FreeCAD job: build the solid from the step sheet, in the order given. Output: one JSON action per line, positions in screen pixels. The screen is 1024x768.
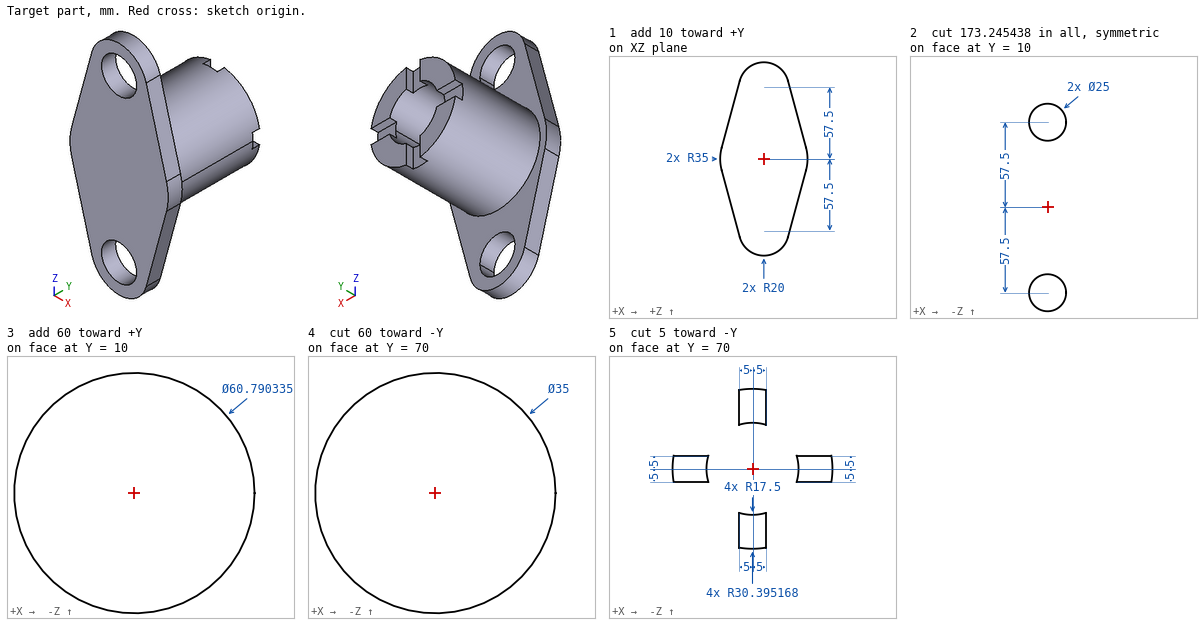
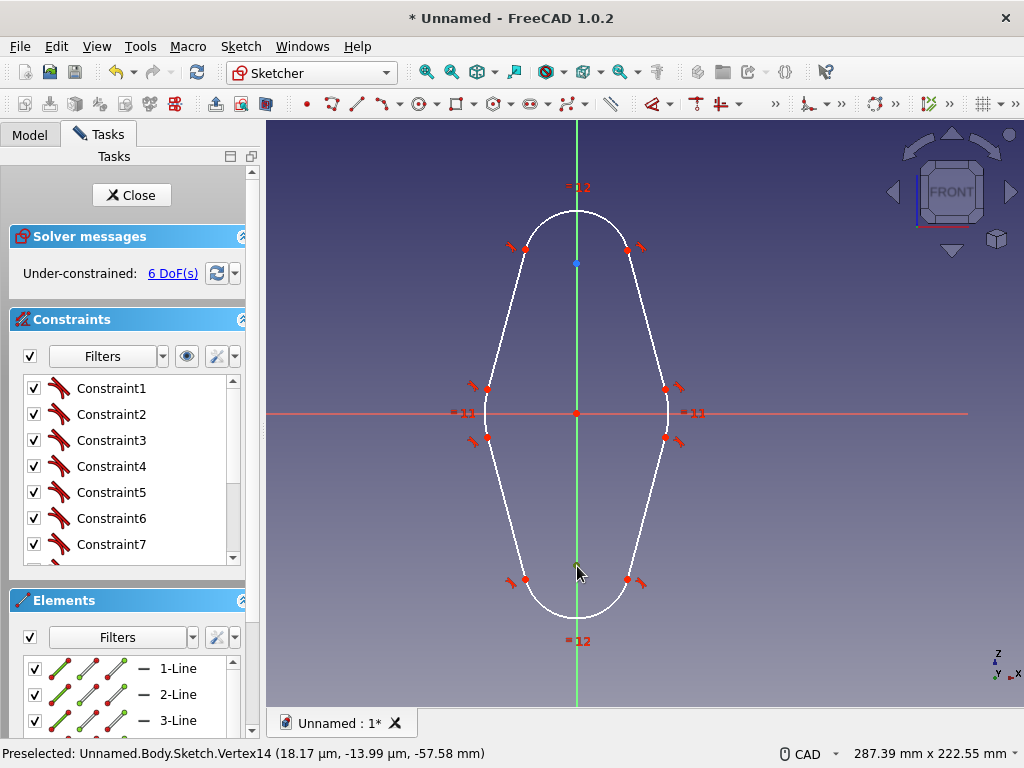
{"action": "left_click", "coordinate": [577, 527]}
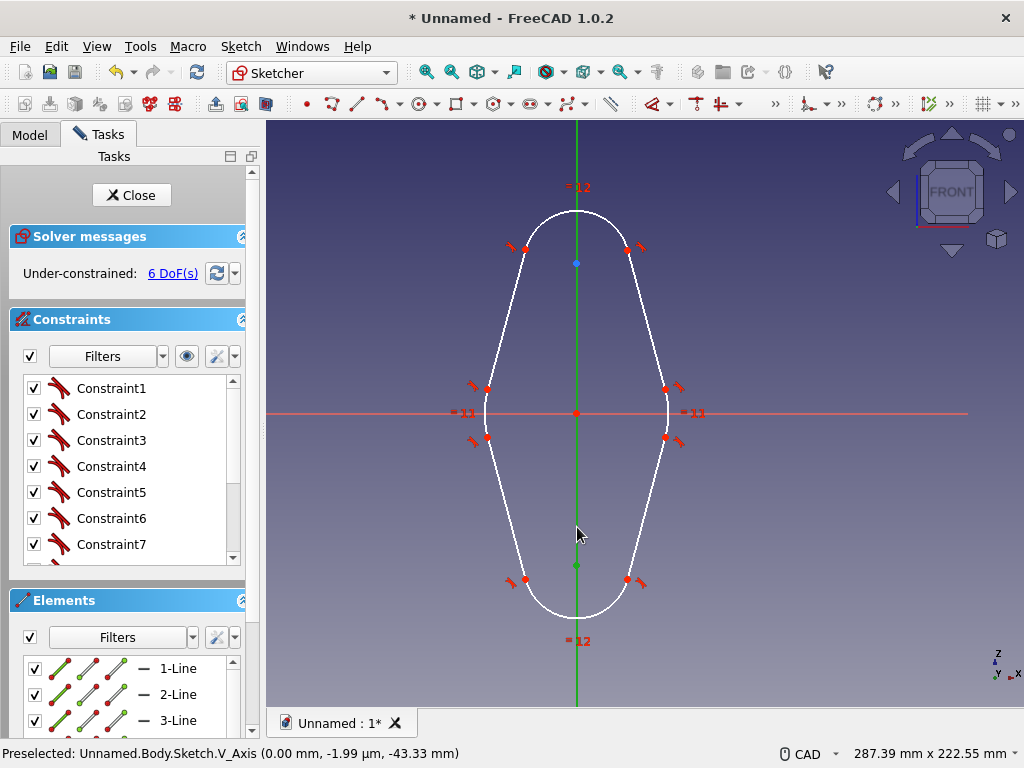
{"action": "key", "text": "c"}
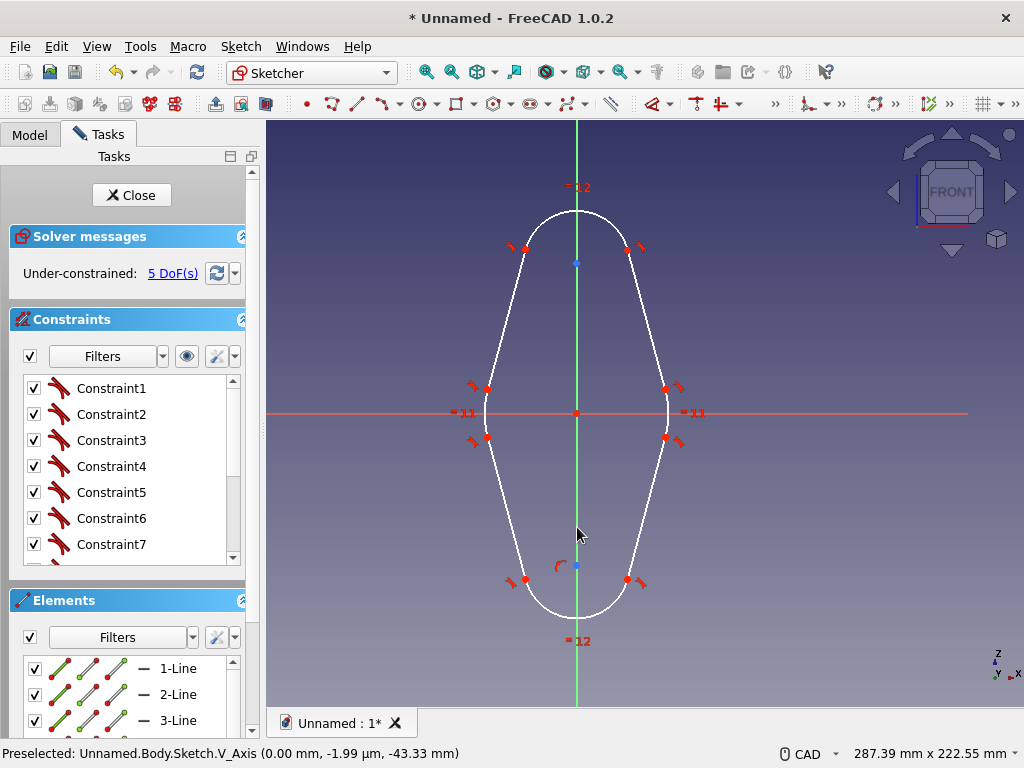
{"action": "left_click", "coordinate": [577, 264]}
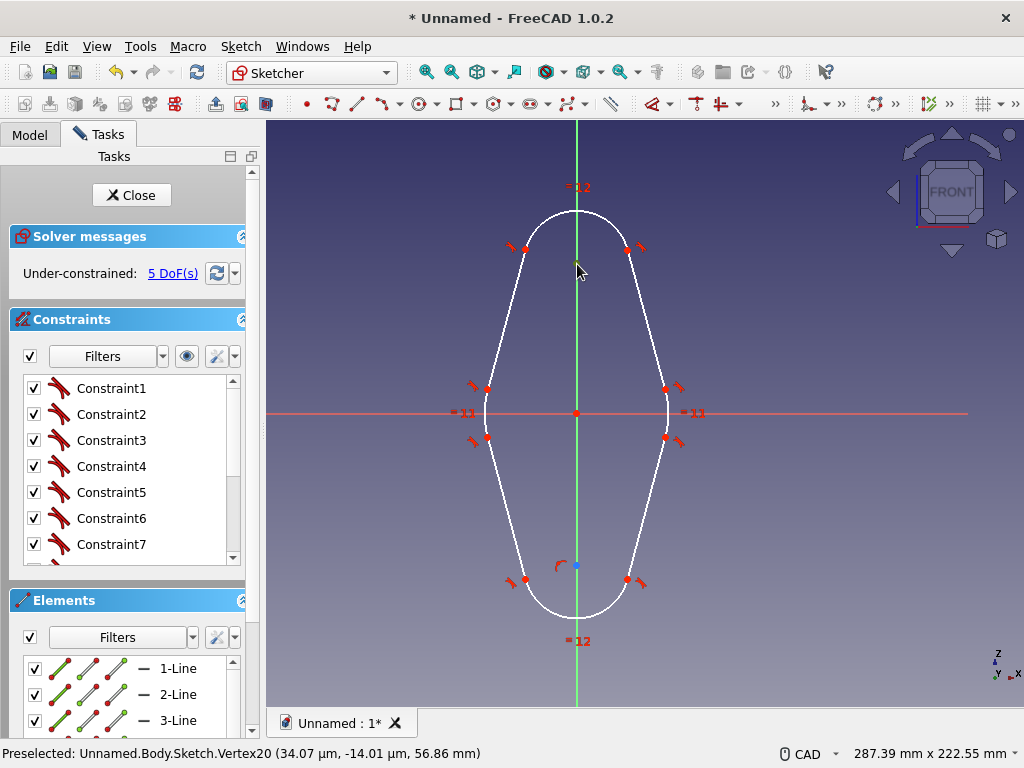
{"action": "left_click", "coordinate": [577, 527]}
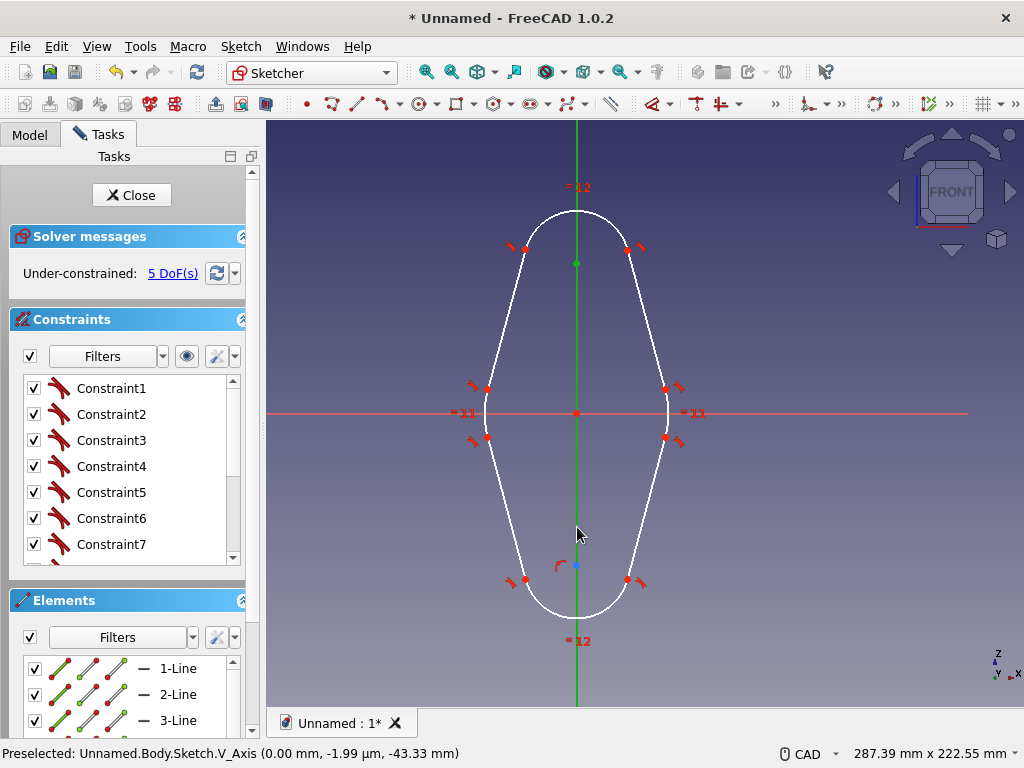
{"action": "left_click", "coordinate": [696, 104]}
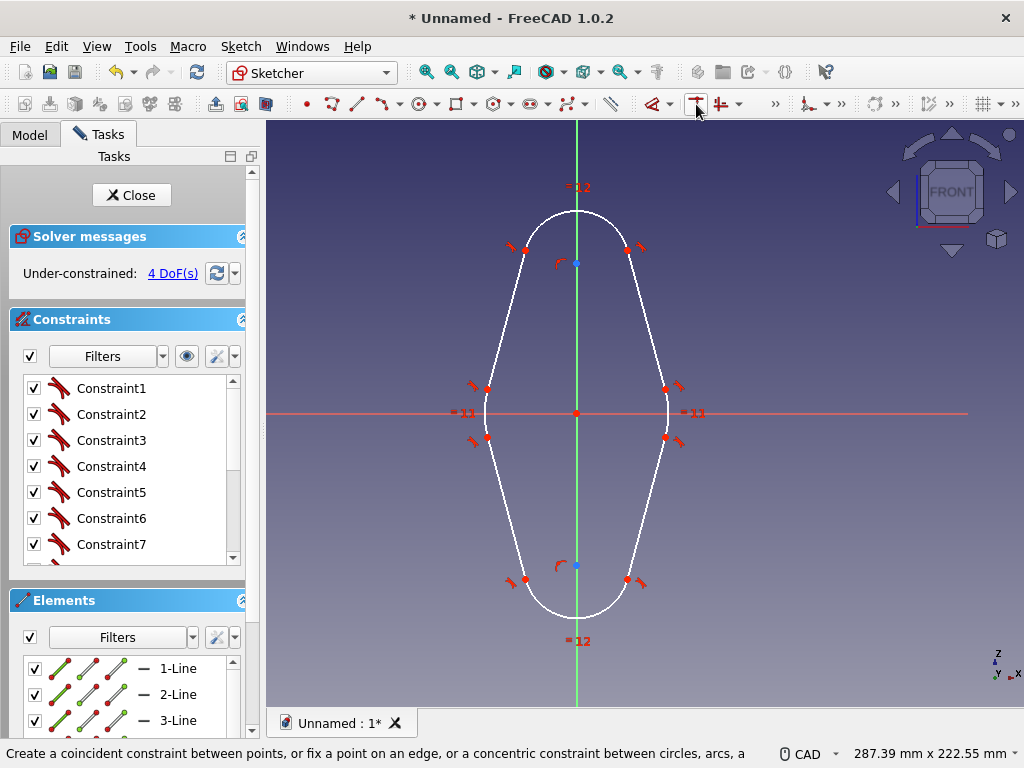
{"action": "scroll", "coordinate": [668, 423], "scroll_direction": "up", "scroll_amount": 2}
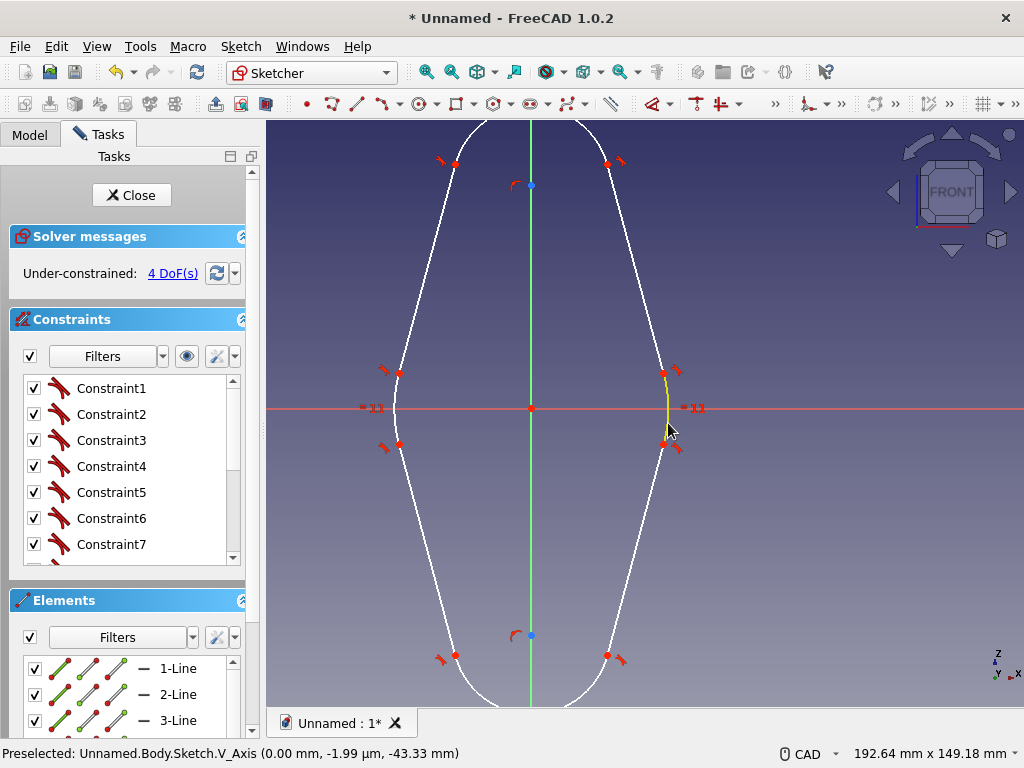
{"action": "left_click", "coordinate": [668, 423]}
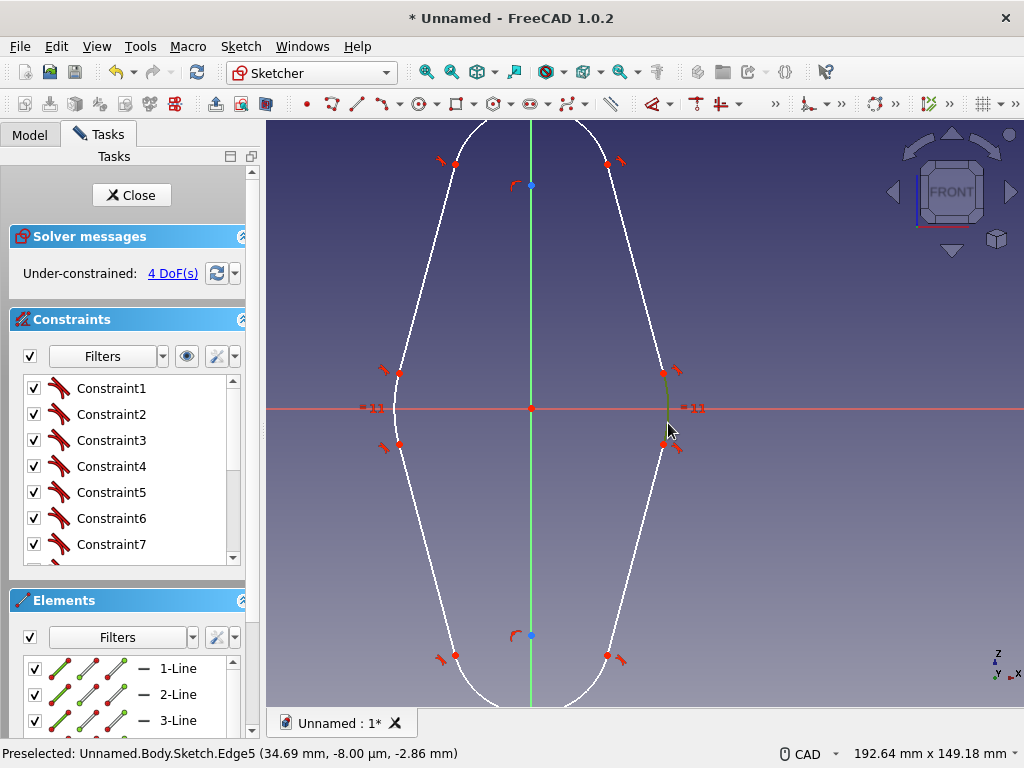
{"action": "key", "text": "k r"}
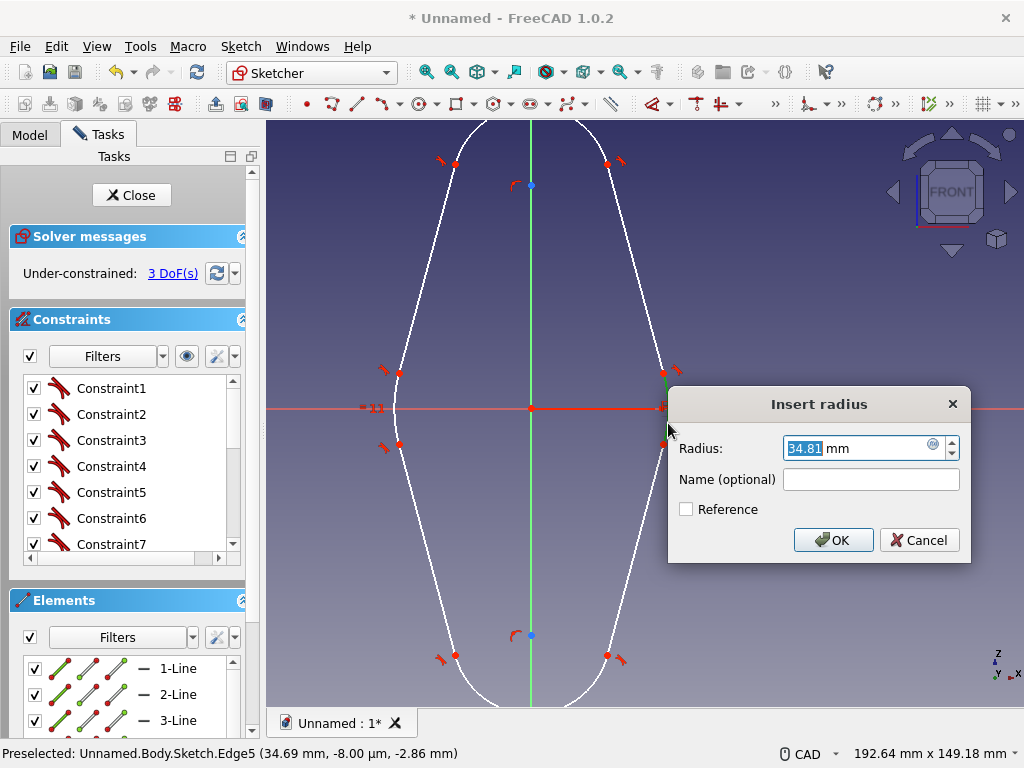
{"action": "type", "text": "35"}
{"action": "key", "text": "Return"}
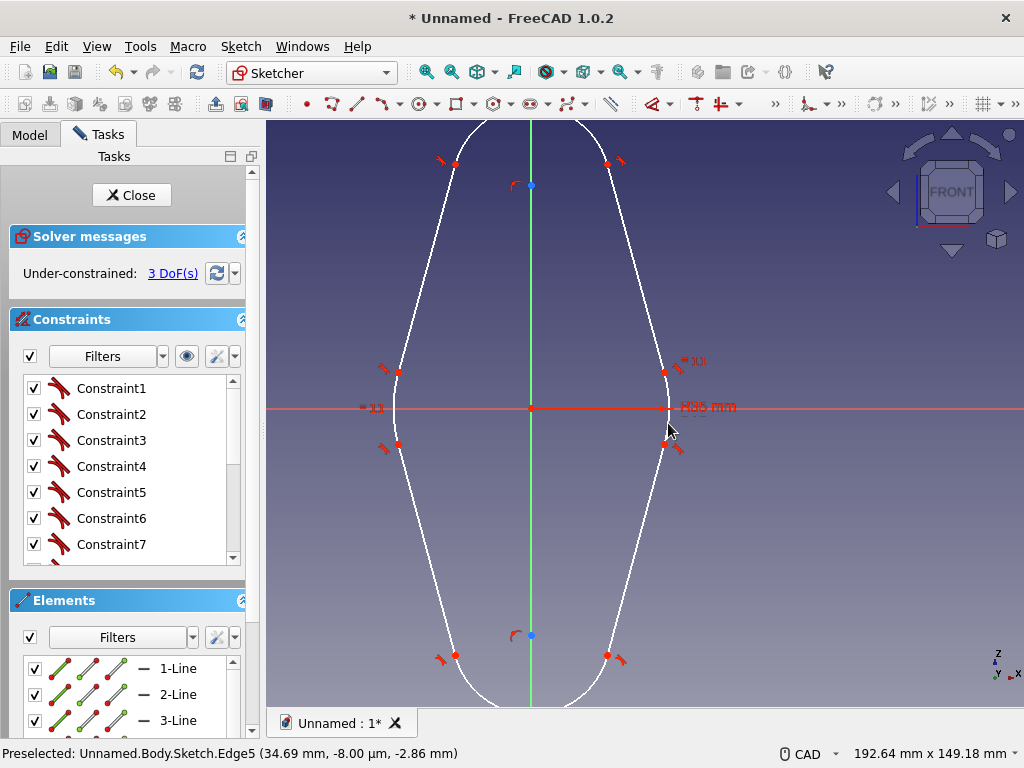
{"action": "scroll", "coordinate": [668, 423], "scroll_direction": "down", "scroll_amount": 2}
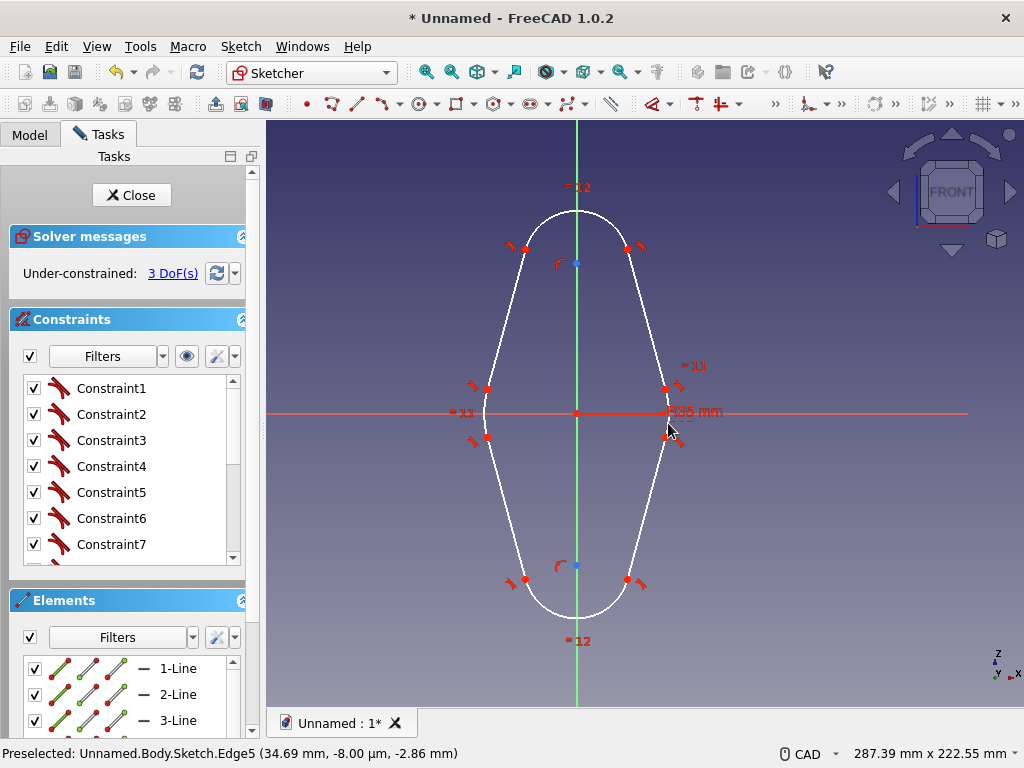
{"action": "left_click", "coordinate": [550, 611]}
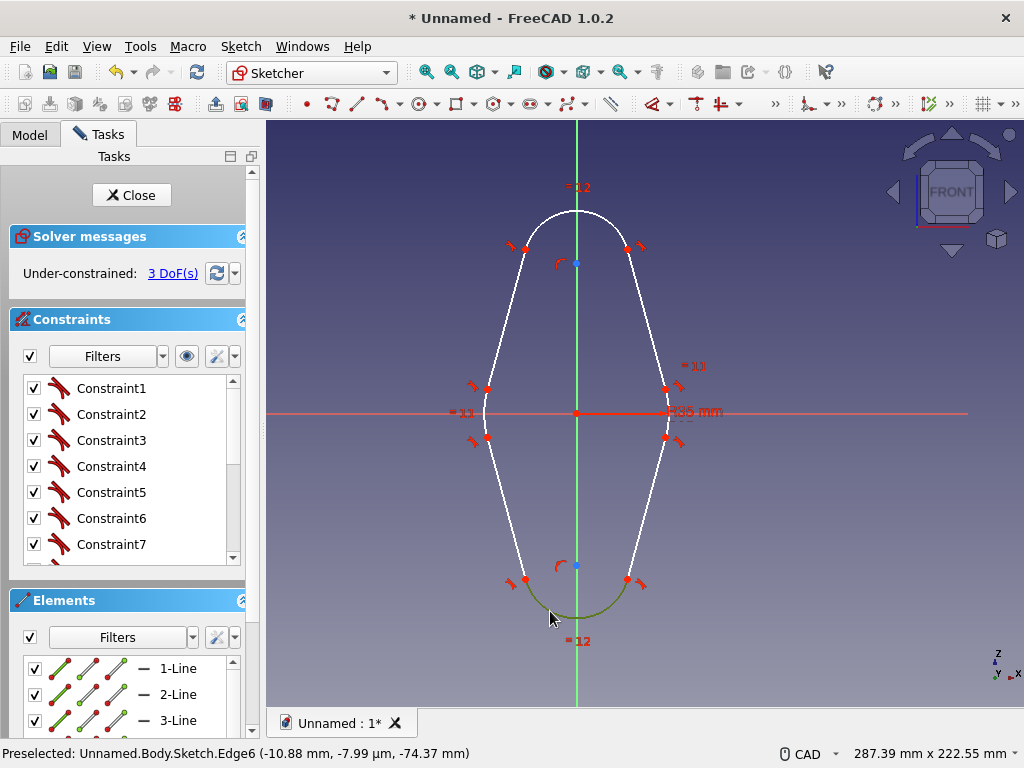
{"action": "left_click", "coordinate": [670, 104]}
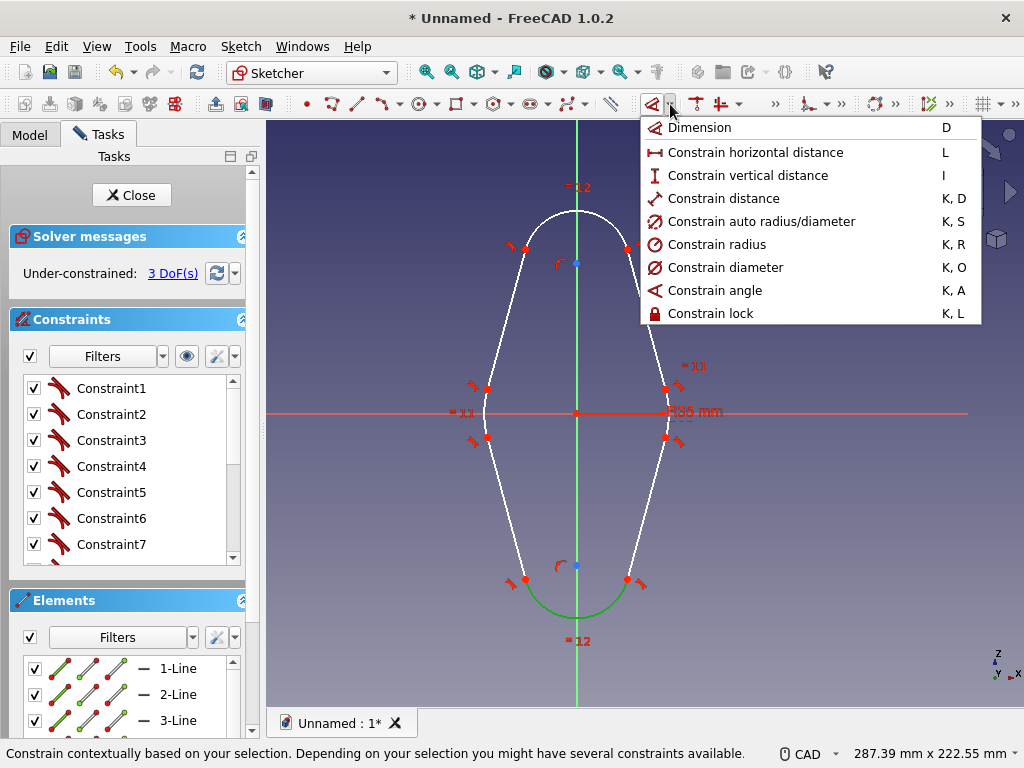
{"action": "left_click", "coordinate": [811, 244]}